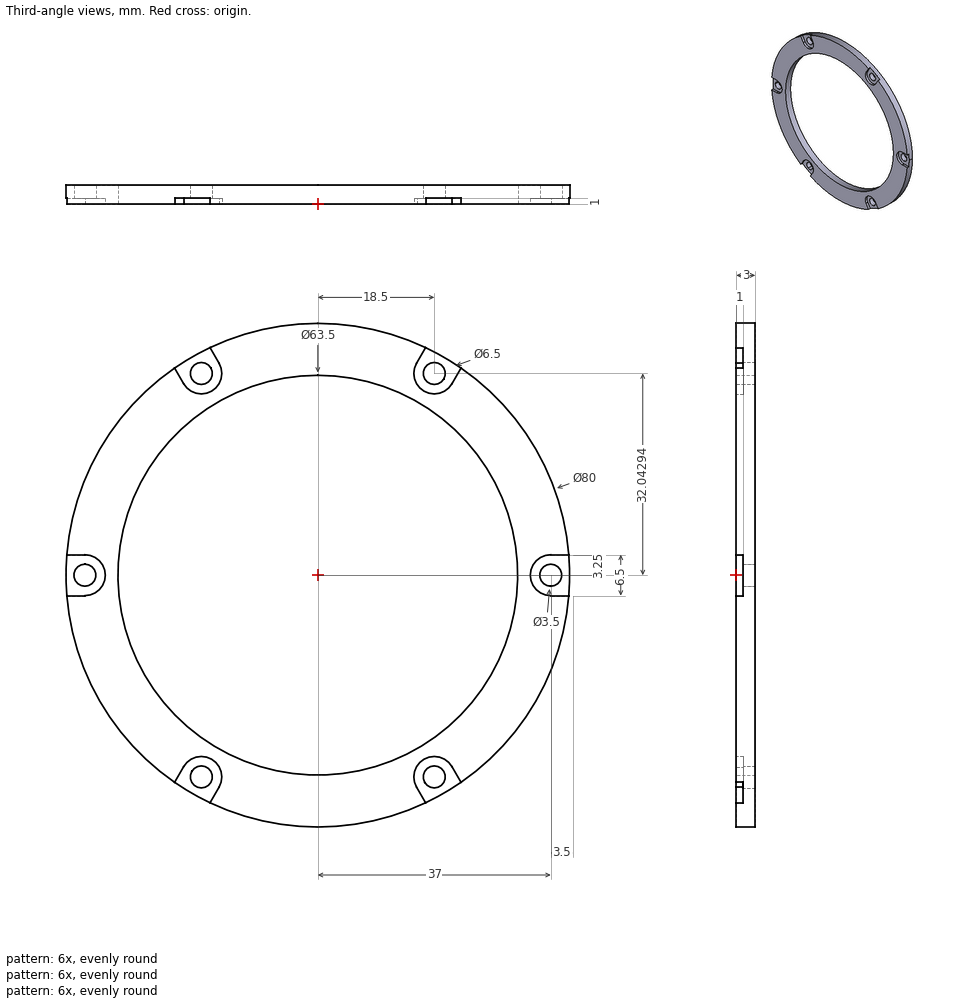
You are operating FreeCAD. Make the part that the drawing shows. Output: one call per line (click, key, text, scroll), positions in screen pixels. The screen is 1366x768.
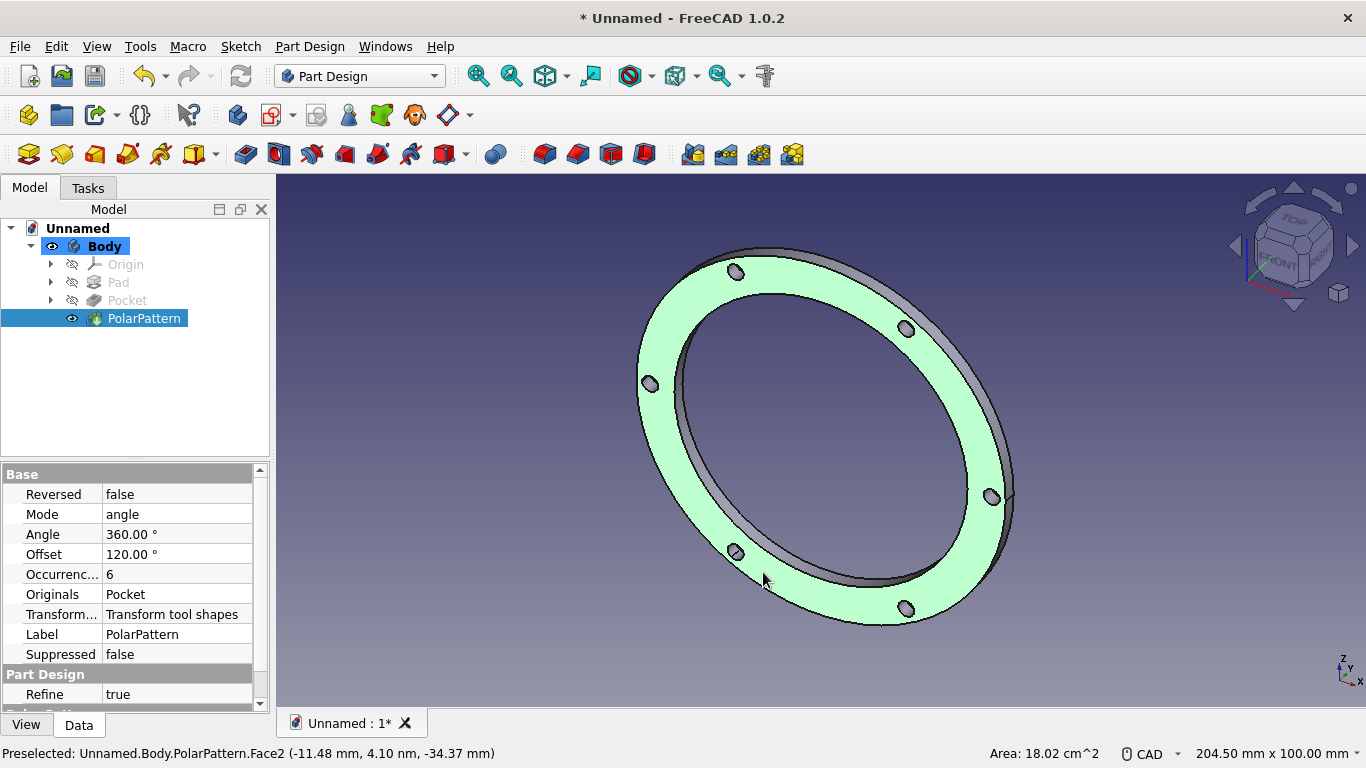
click(270, 116)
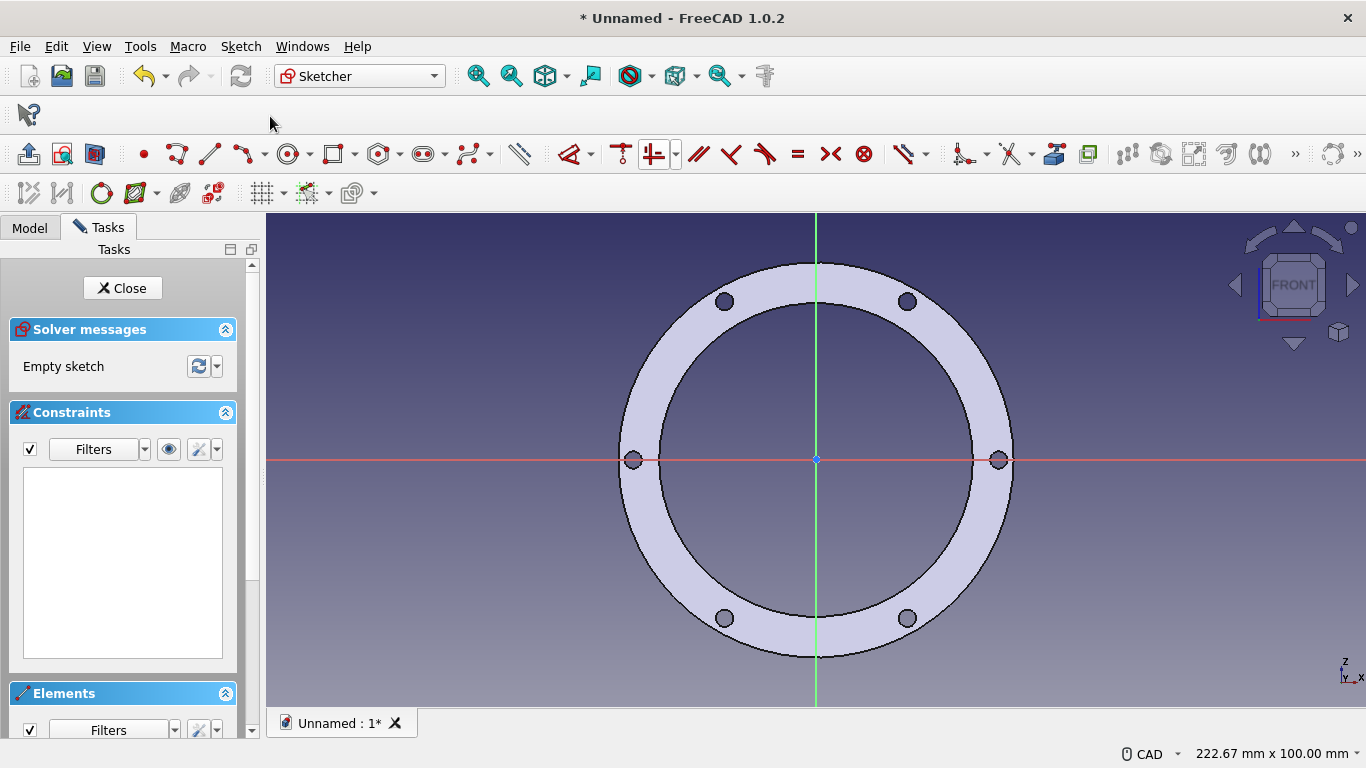
scroll(927, 282, up, 11)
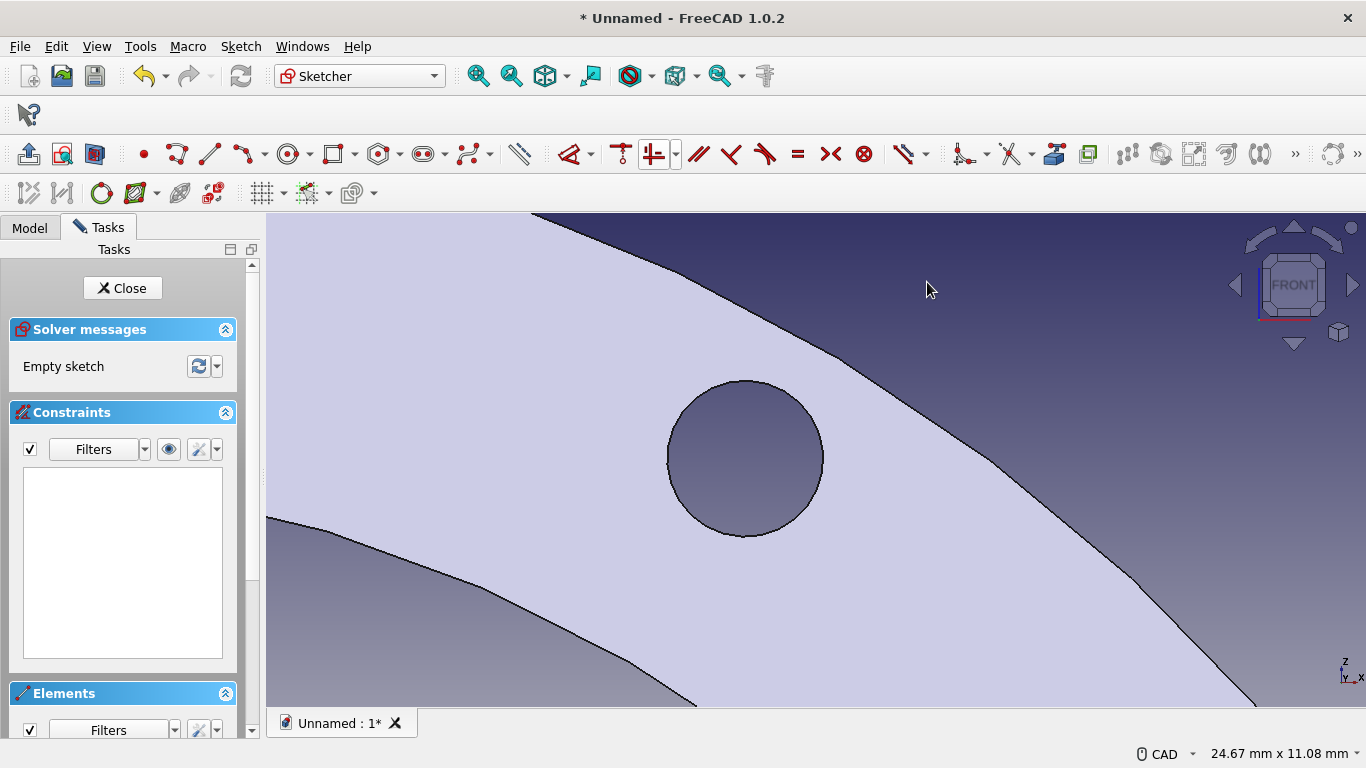
click(288, 154)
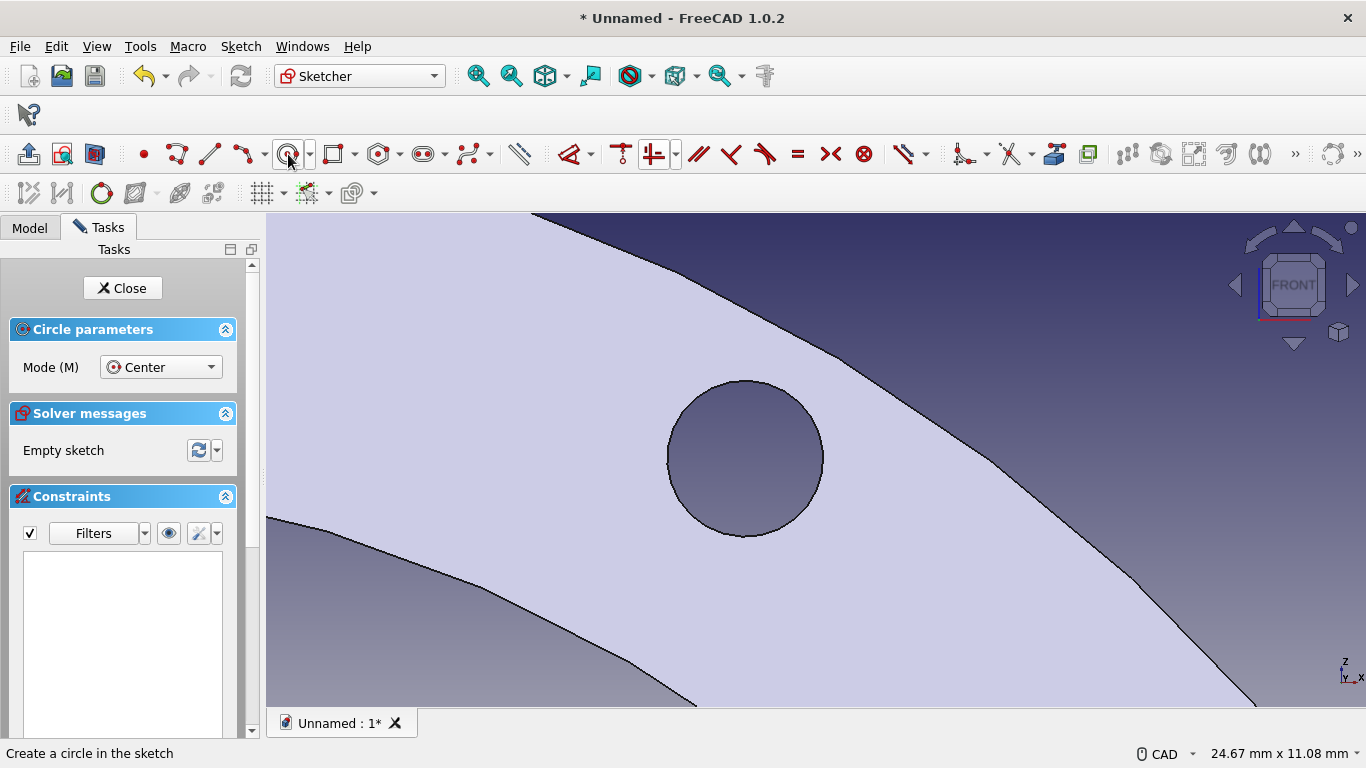
click(745, 459)
move(848, 356)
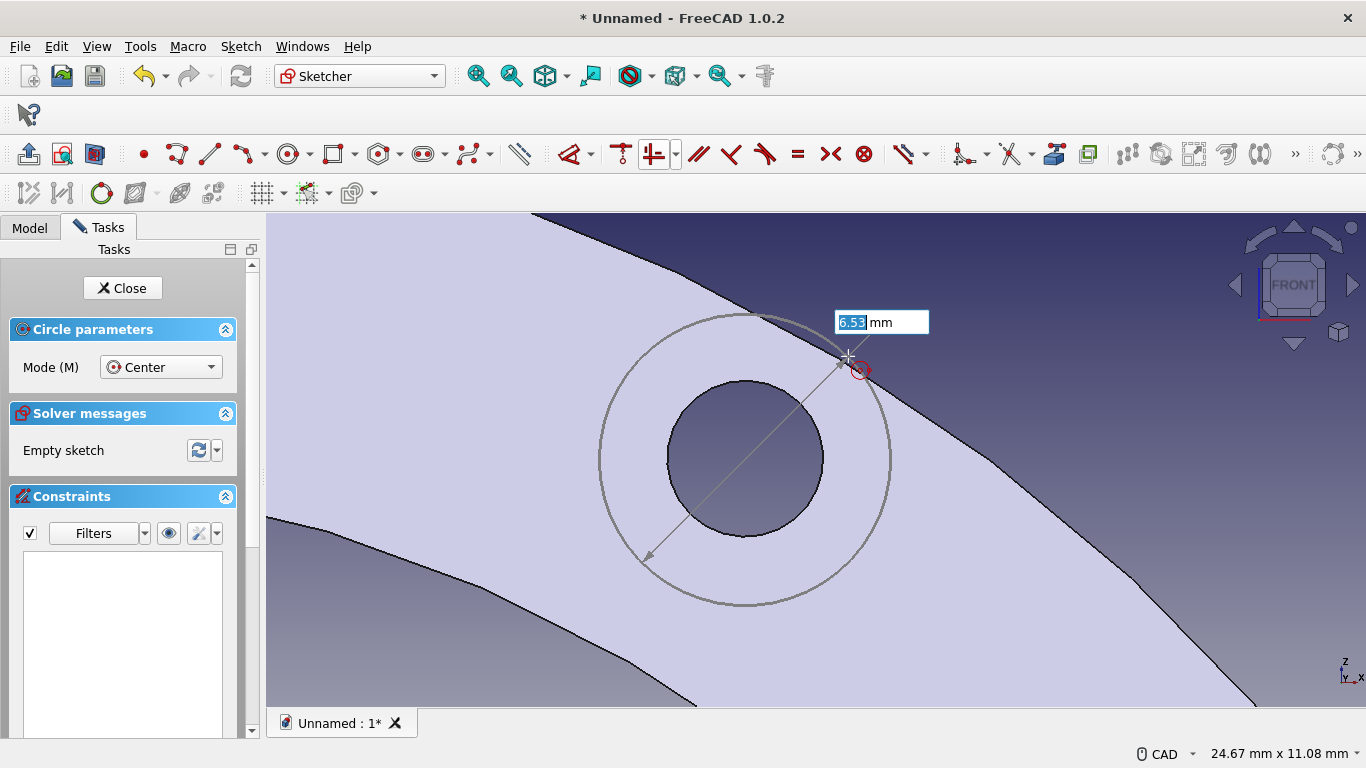
text(6.5)
key(Return)
key(Escape)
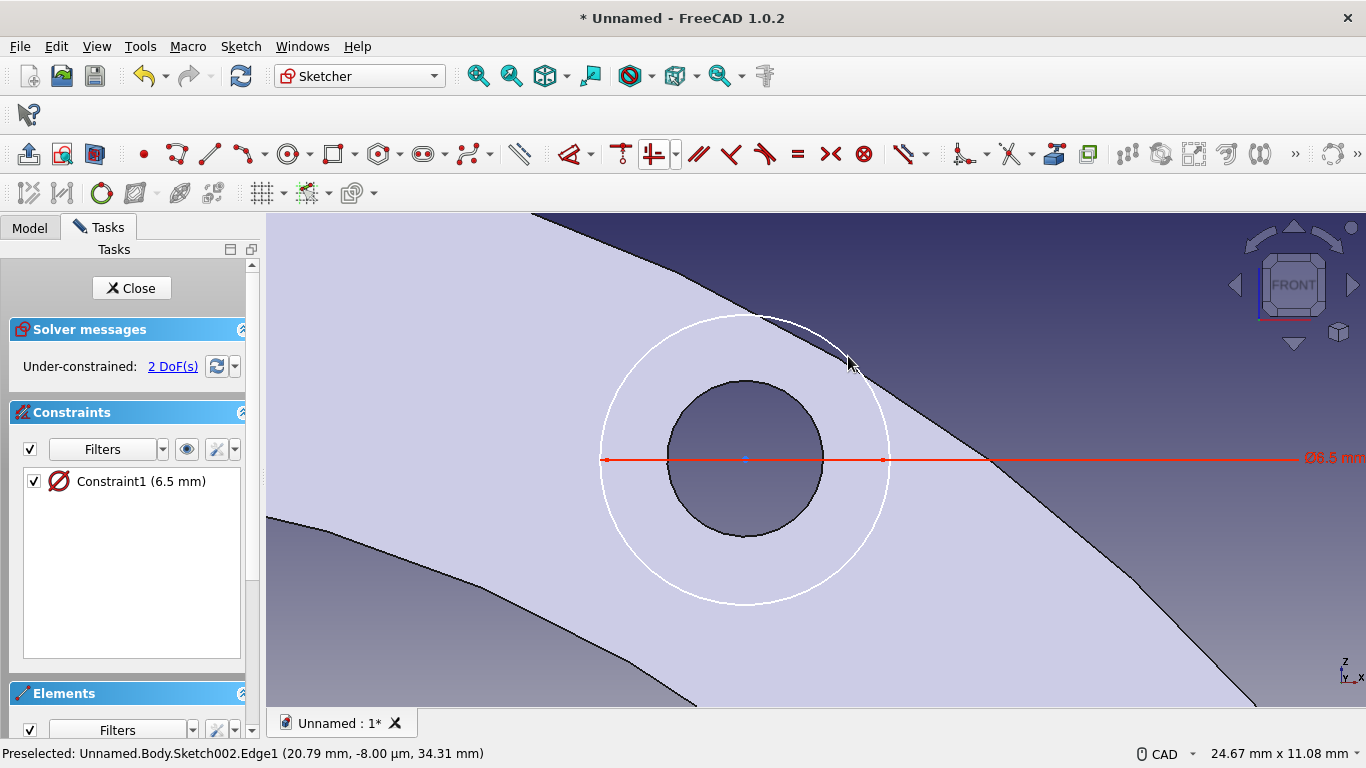
click(568, 154)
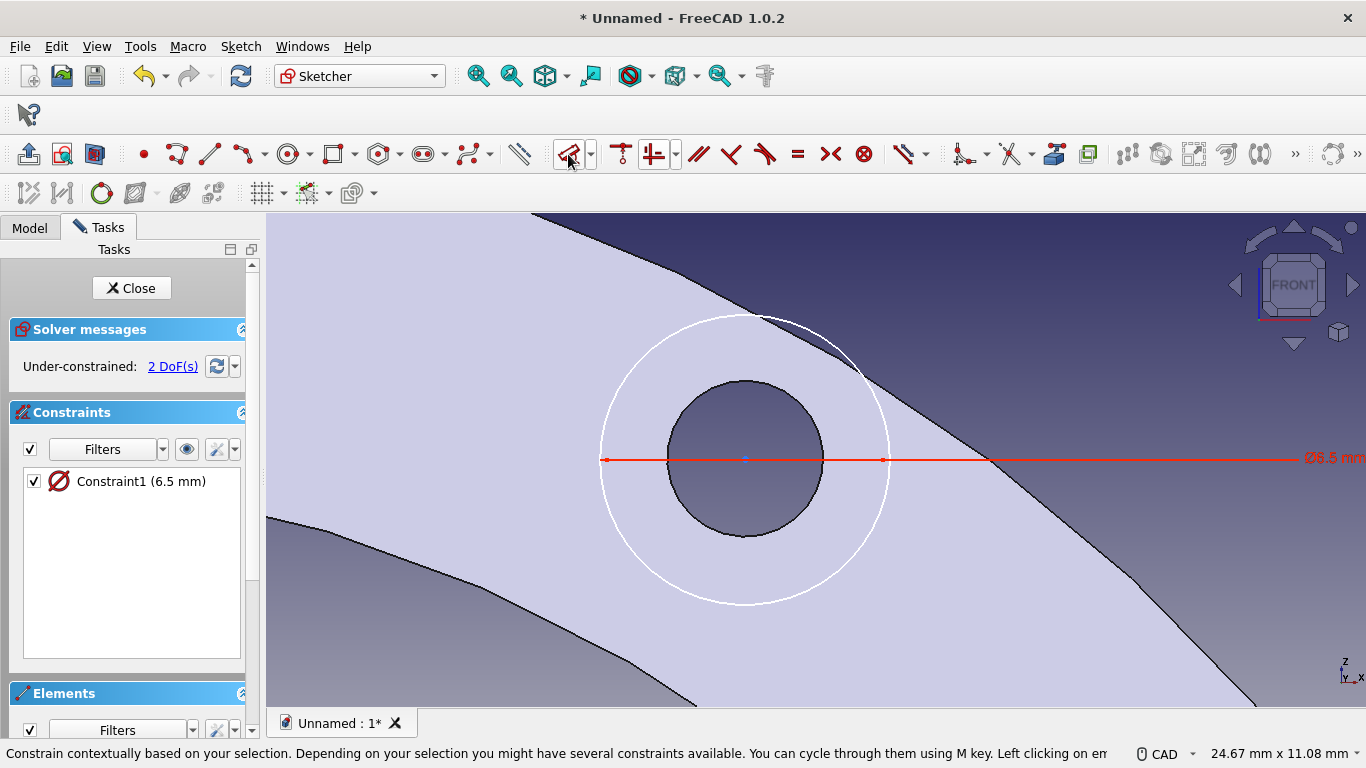
click(745, 460)
click(519, 426)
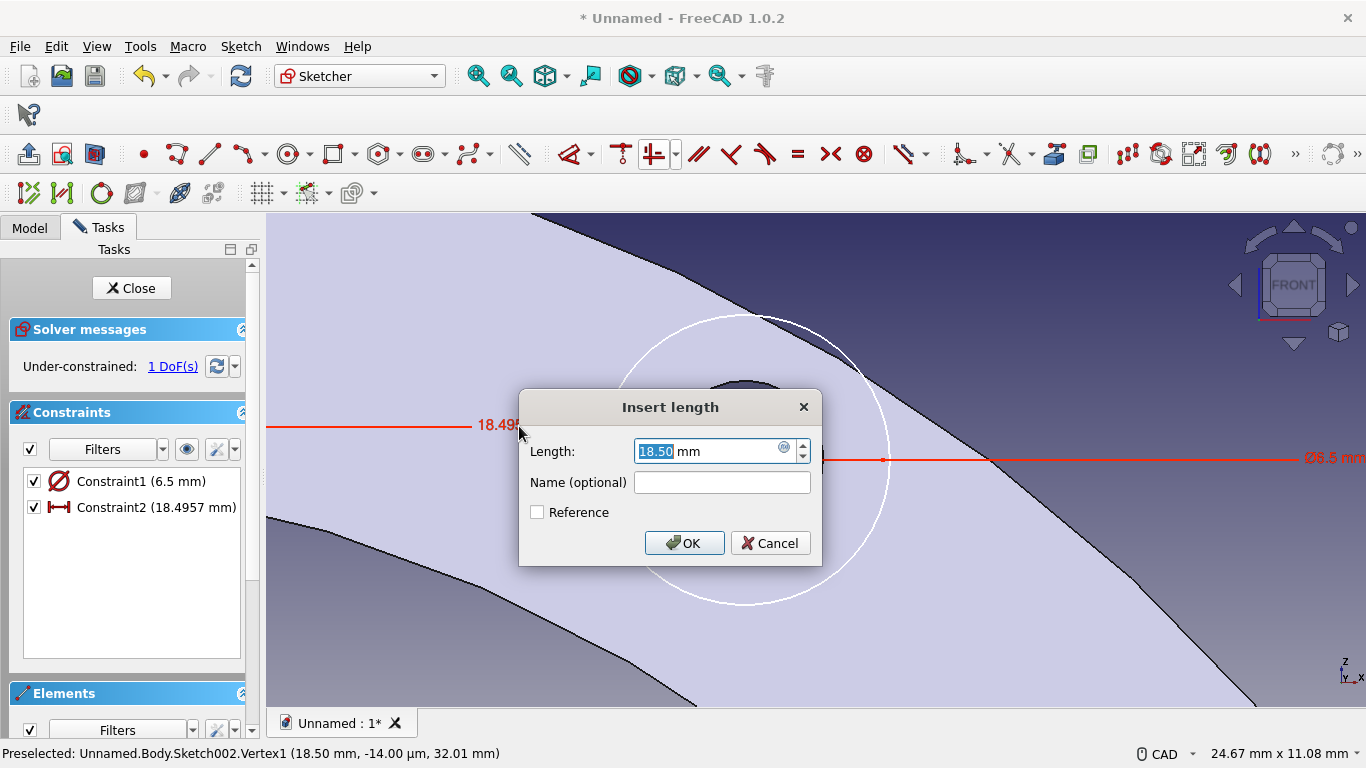
text(18.5)
key(Return)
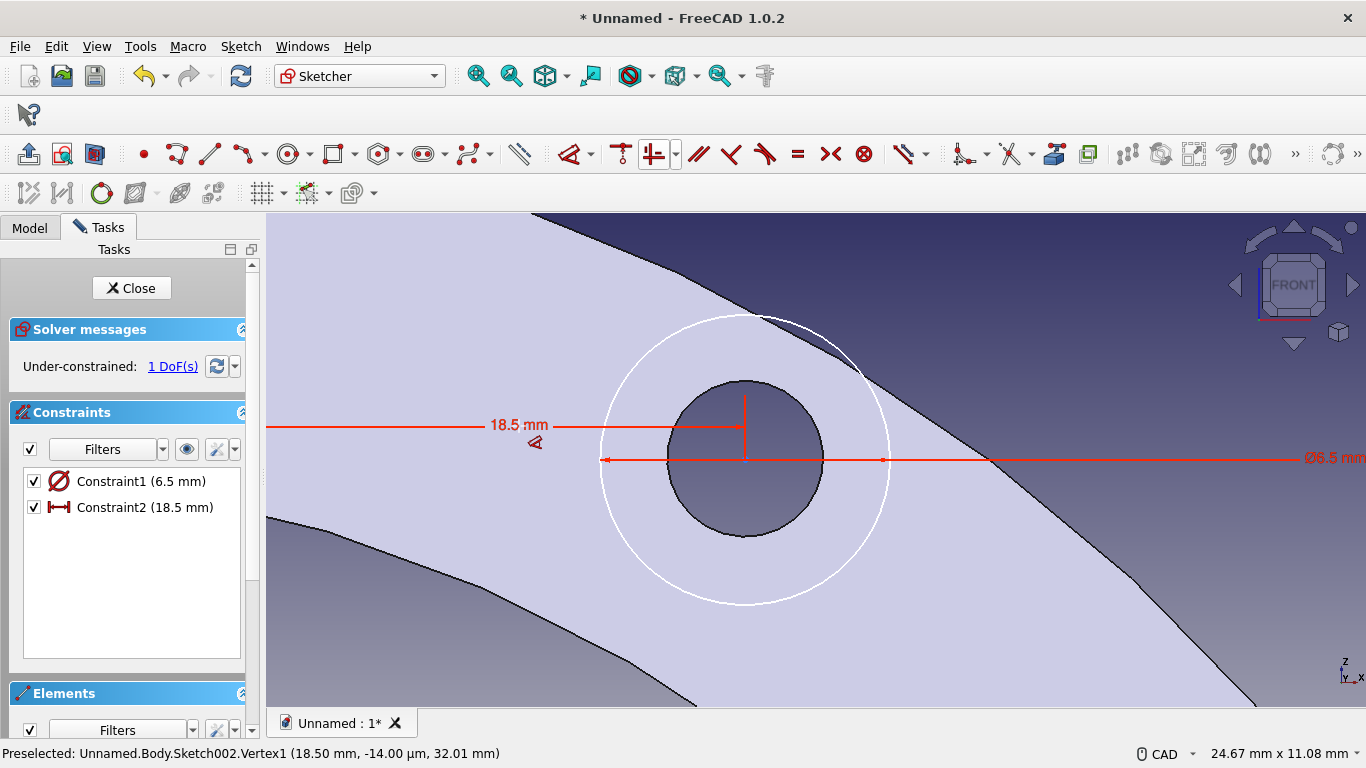
click(745, 460)
click(779, 570)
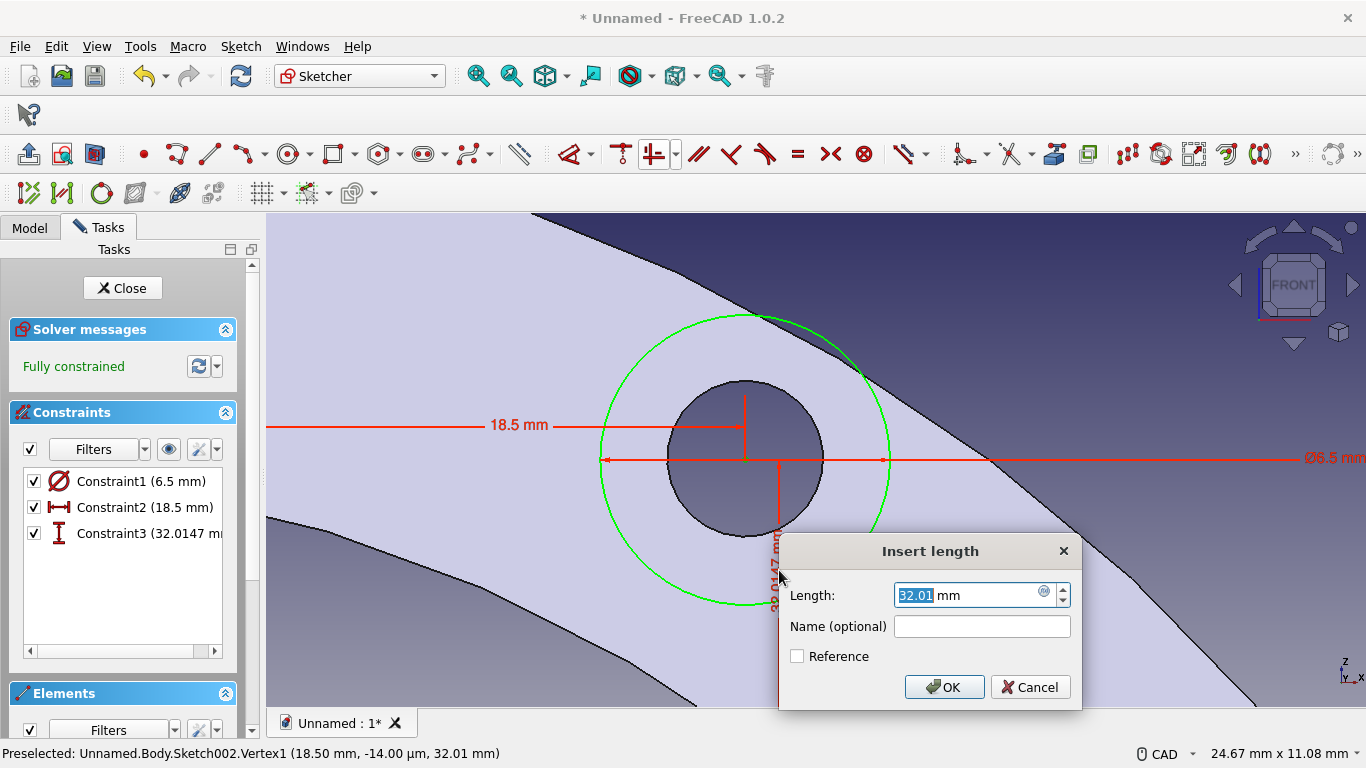
text(32.04294)
key(Return)
key(Escape)